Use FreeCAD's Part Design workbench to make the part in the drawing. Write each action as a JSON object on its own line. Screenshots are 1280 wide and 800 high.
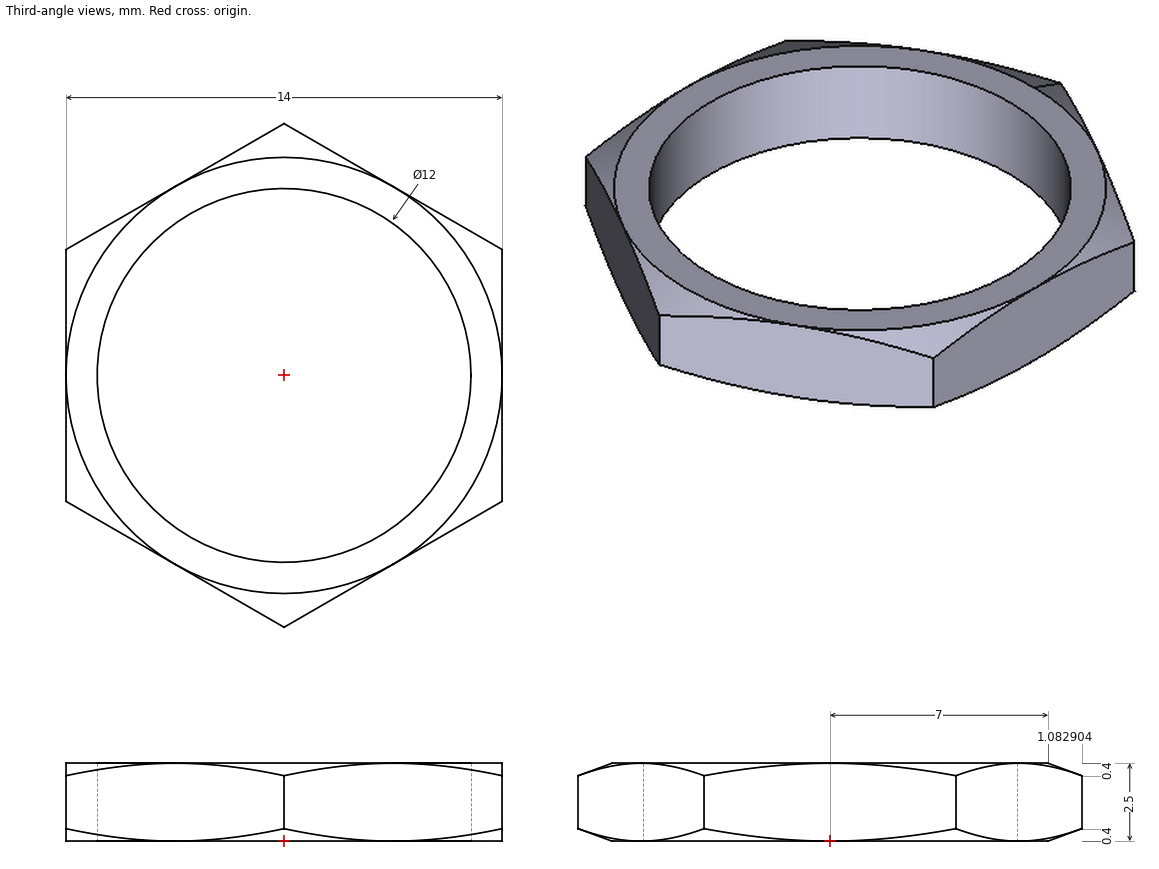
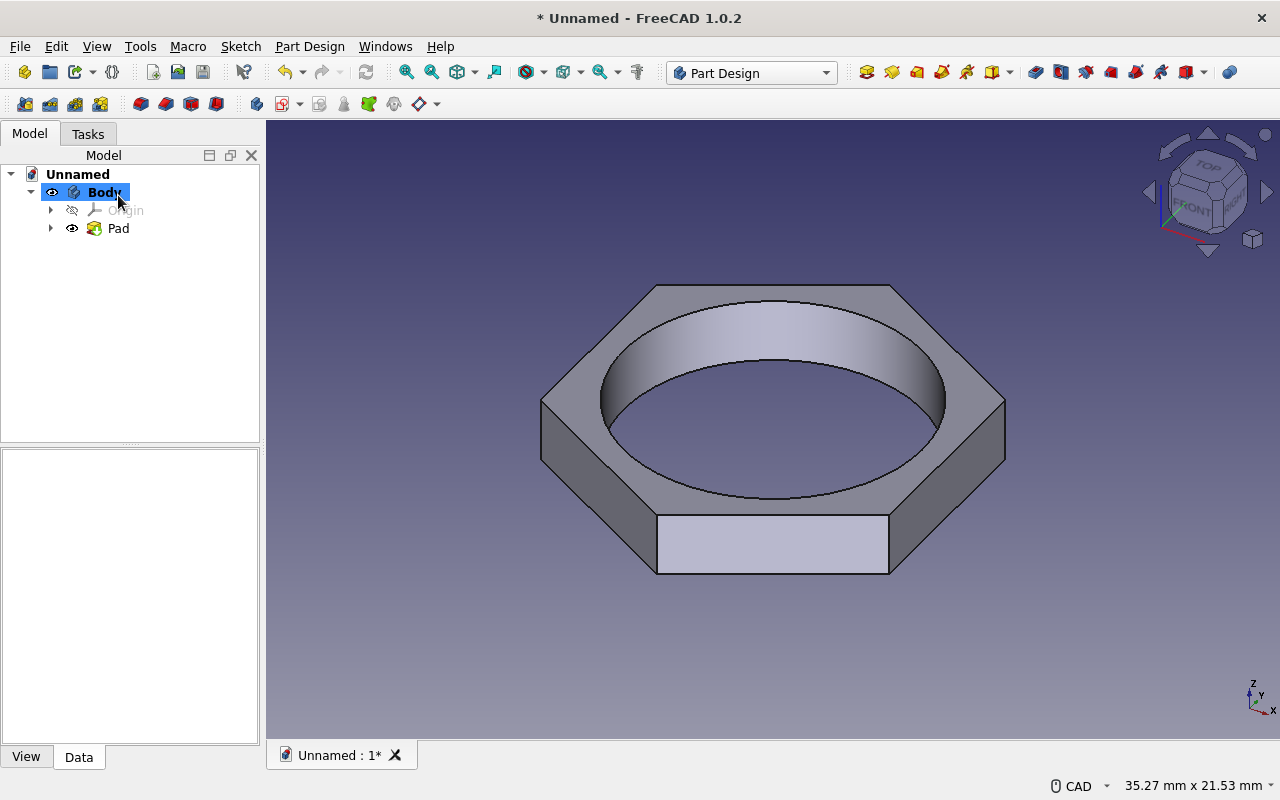
{"action": "left_click", "coordinate": [282, 104]}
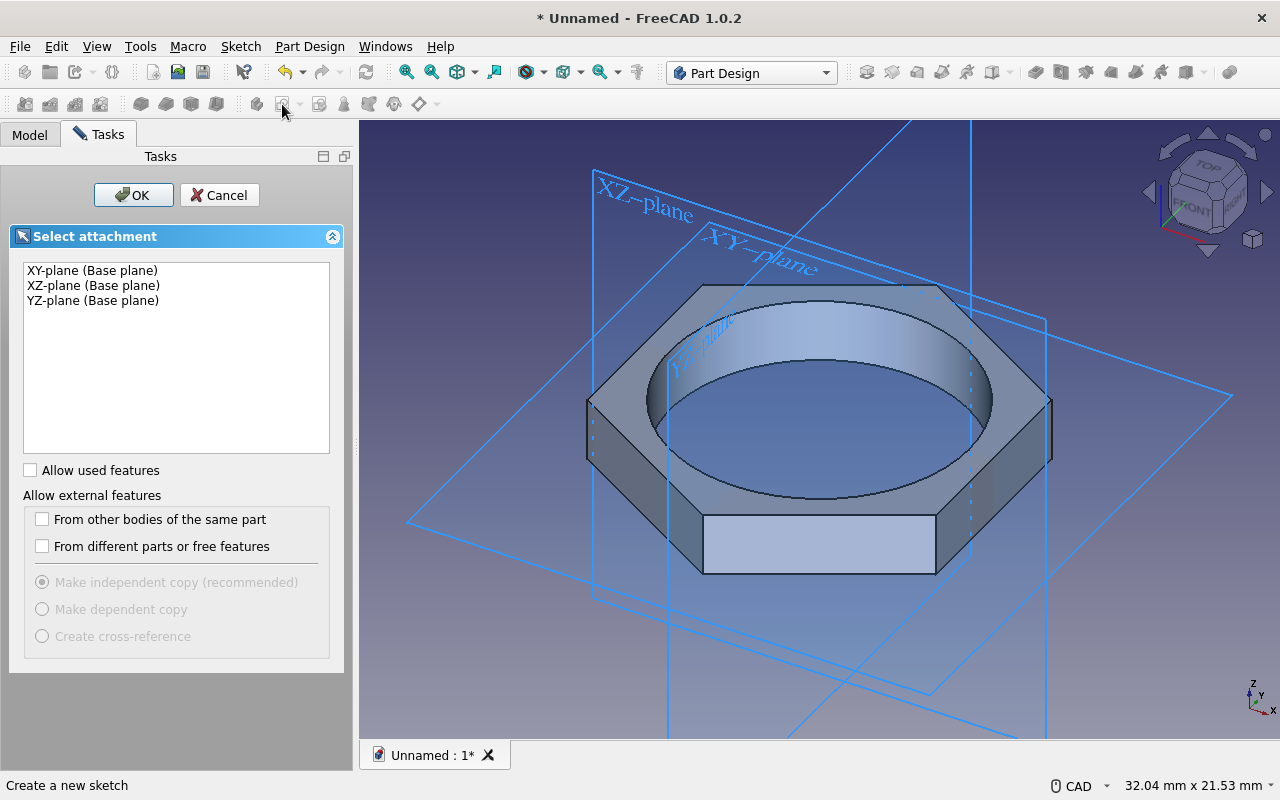
{"action": "left_click", "coordinate": [84, 300]}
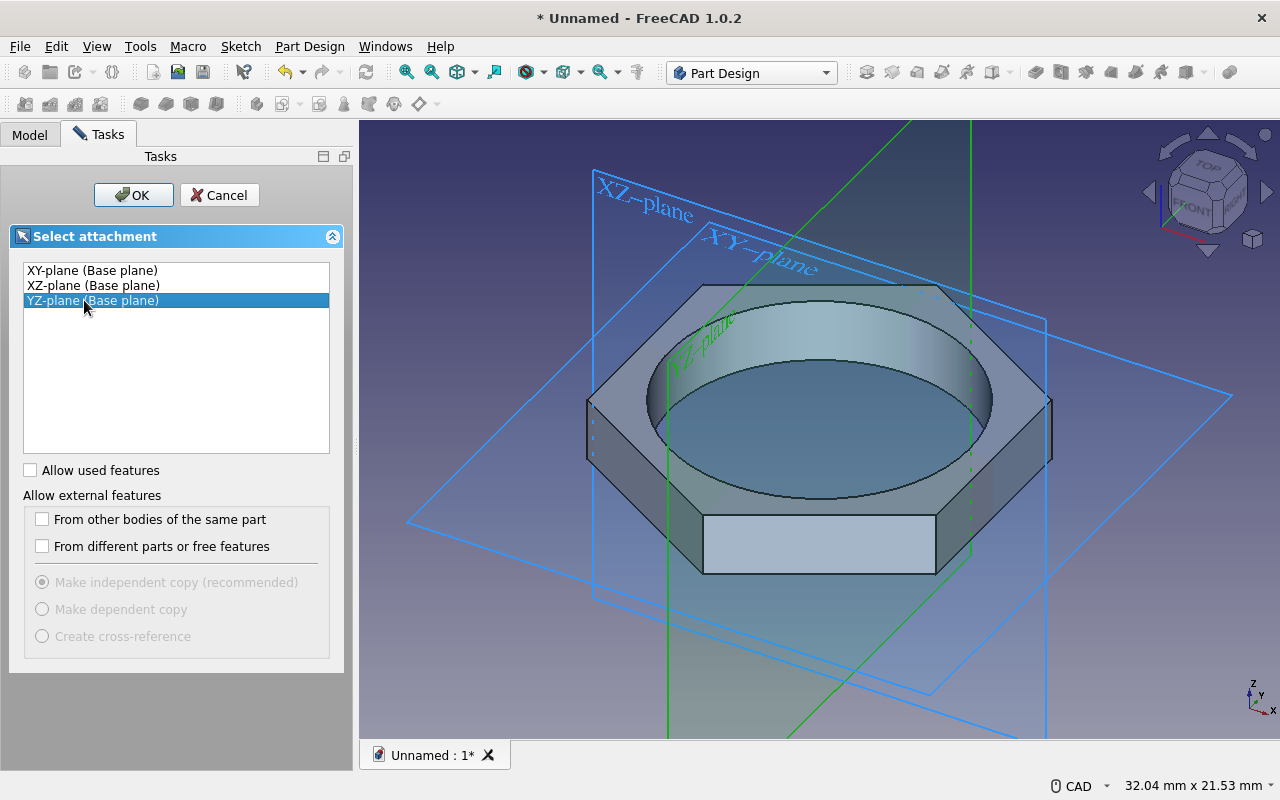
{"action": "left_click", "coordinate": [134, 195]}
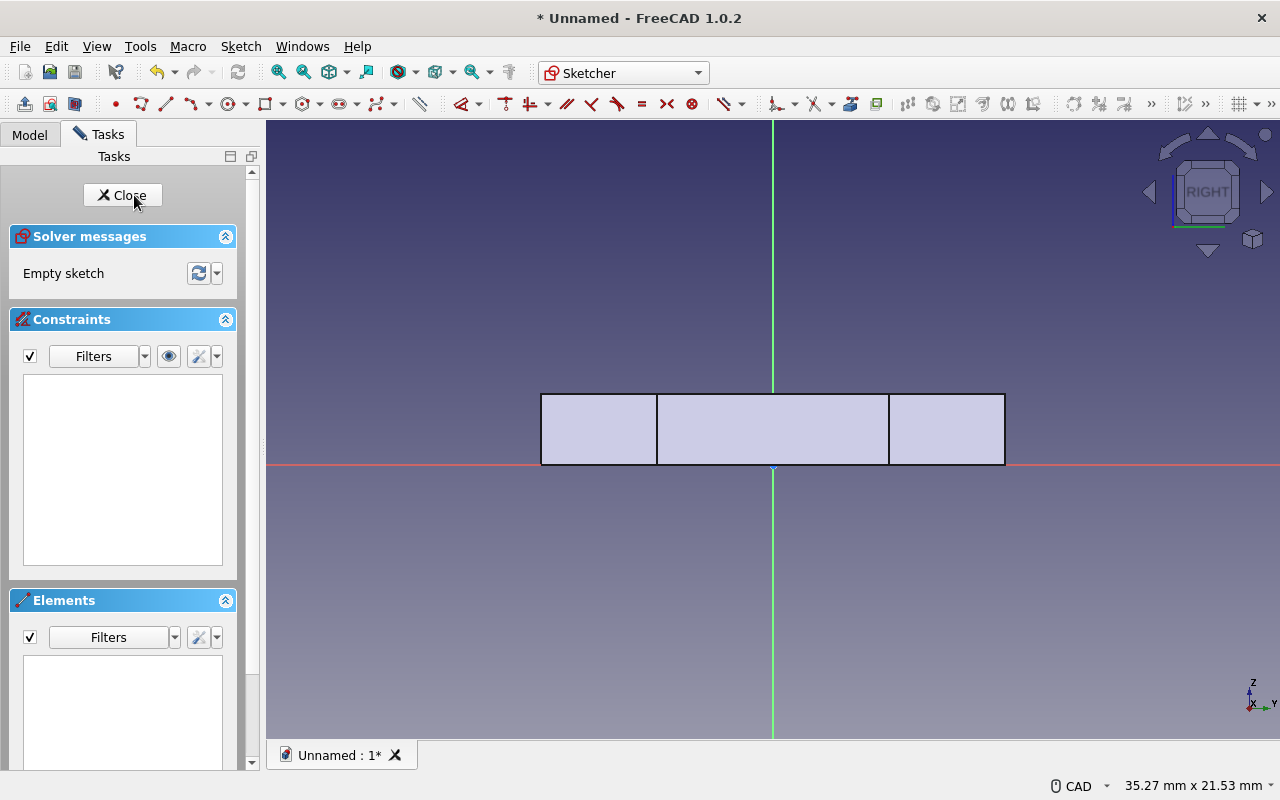
{"action": "key", "text": "q s"}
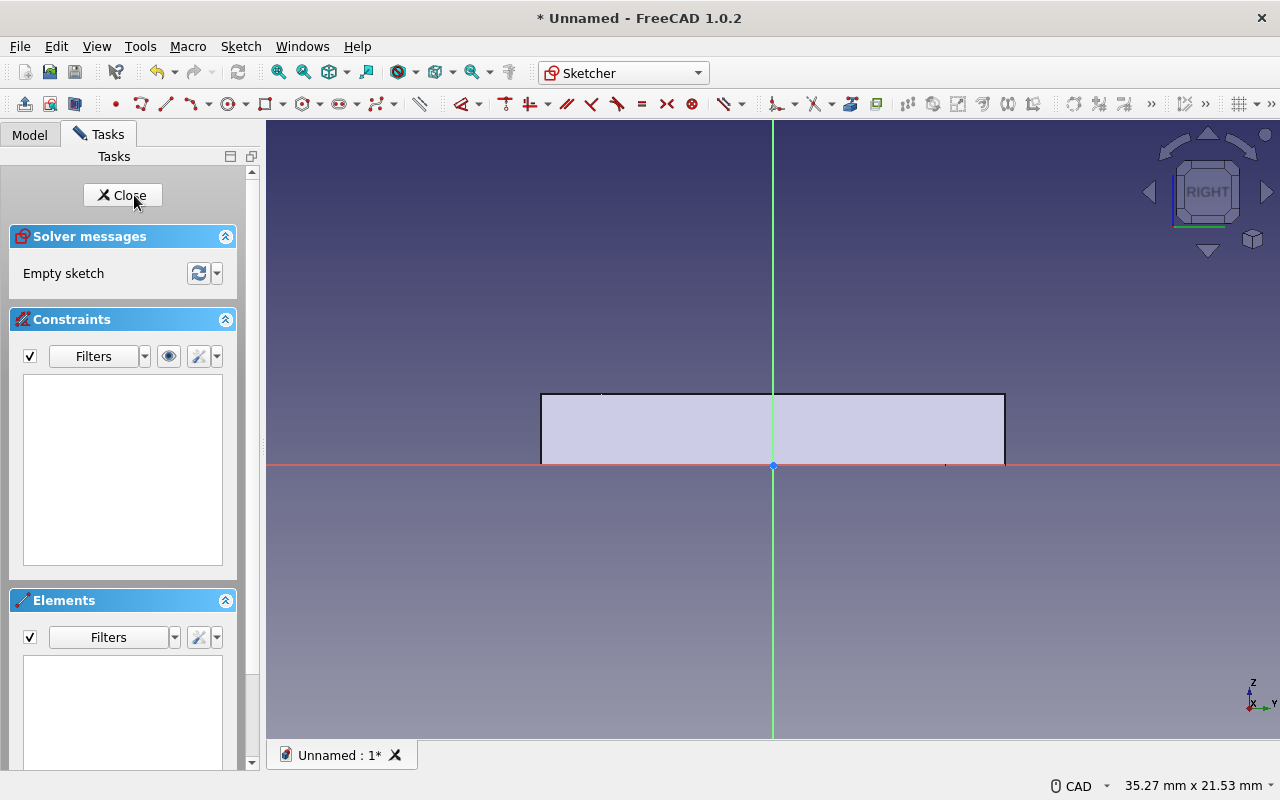
{"action": "scroll", "coordinate": [1046, 430], "scroll_direction": "up", "scroll_amount": 9}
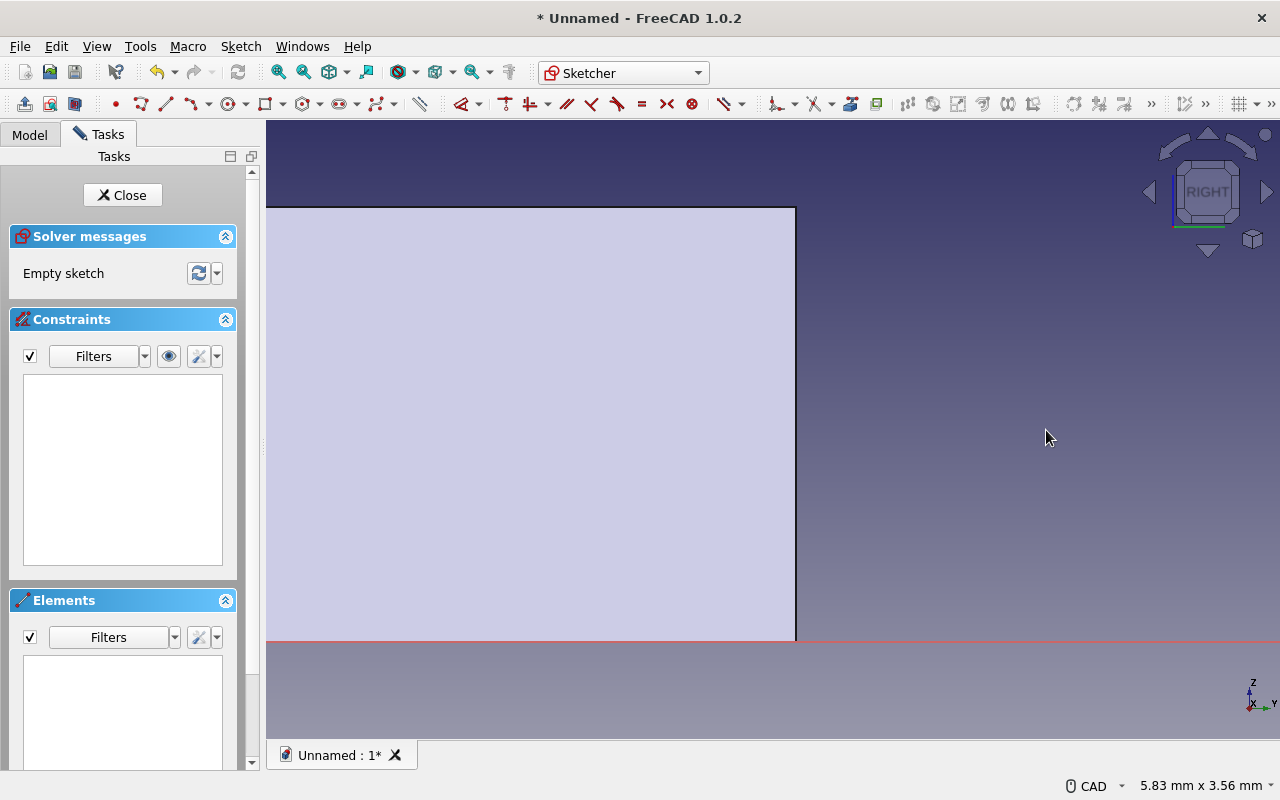
{"action": "key", "text": "g m"}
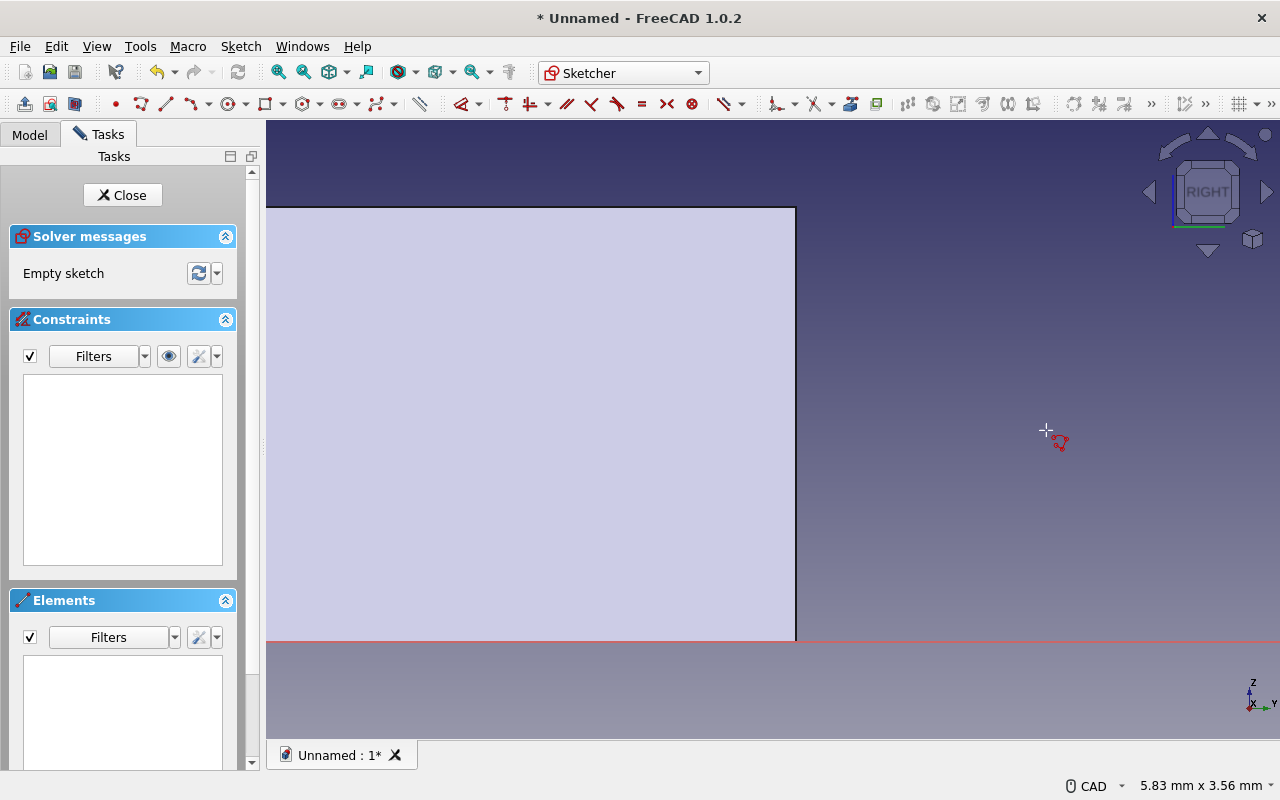
{"action": "left_click", "coordinate": [608, 207]}
{"action": "left_click", "coordinate": [796, 277]}
{"action": "left_click", "coordinate": [796, 207]}
{"action": "left_click", "coordinate": [608, 208]}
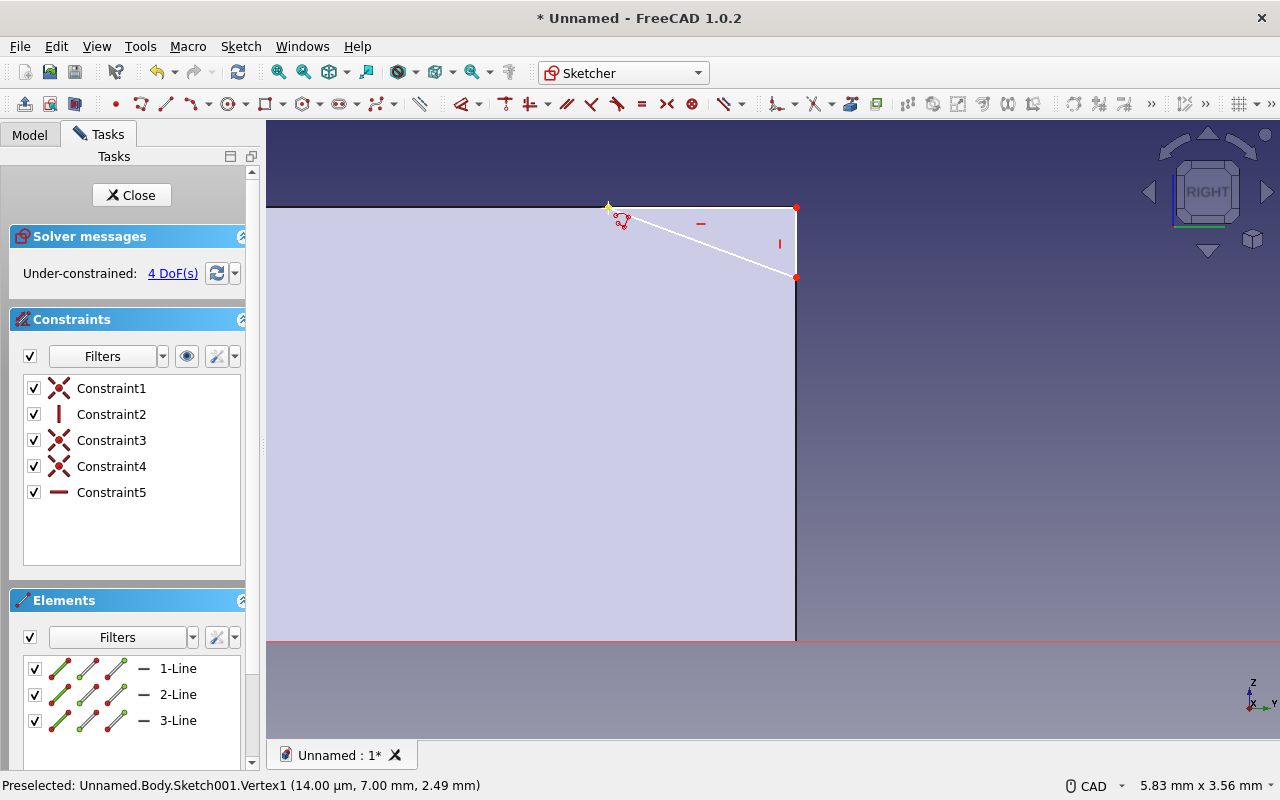
{"action": "left_click", "coordinate": [608, 642]}
{"action": "left_click", "coordinate": [796, 633]}
{"action": "left_click", "coordinate": [796, 572]}
{"action": "left_click", "coordinate": [608, 642]}
{"action": "key", "text": "Escape"}
{"action": "key", "text": "Escape"}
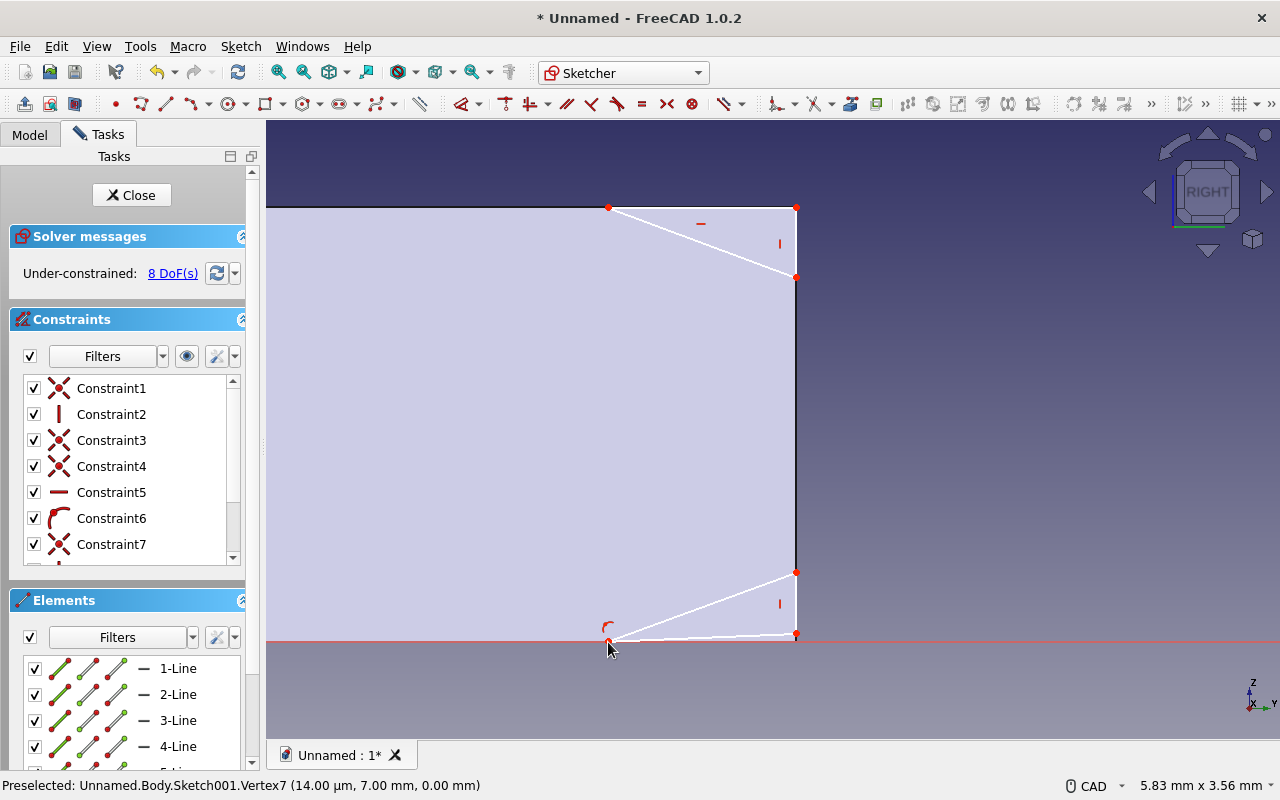
{"action": "left_click", "coordinate": [664, 639]}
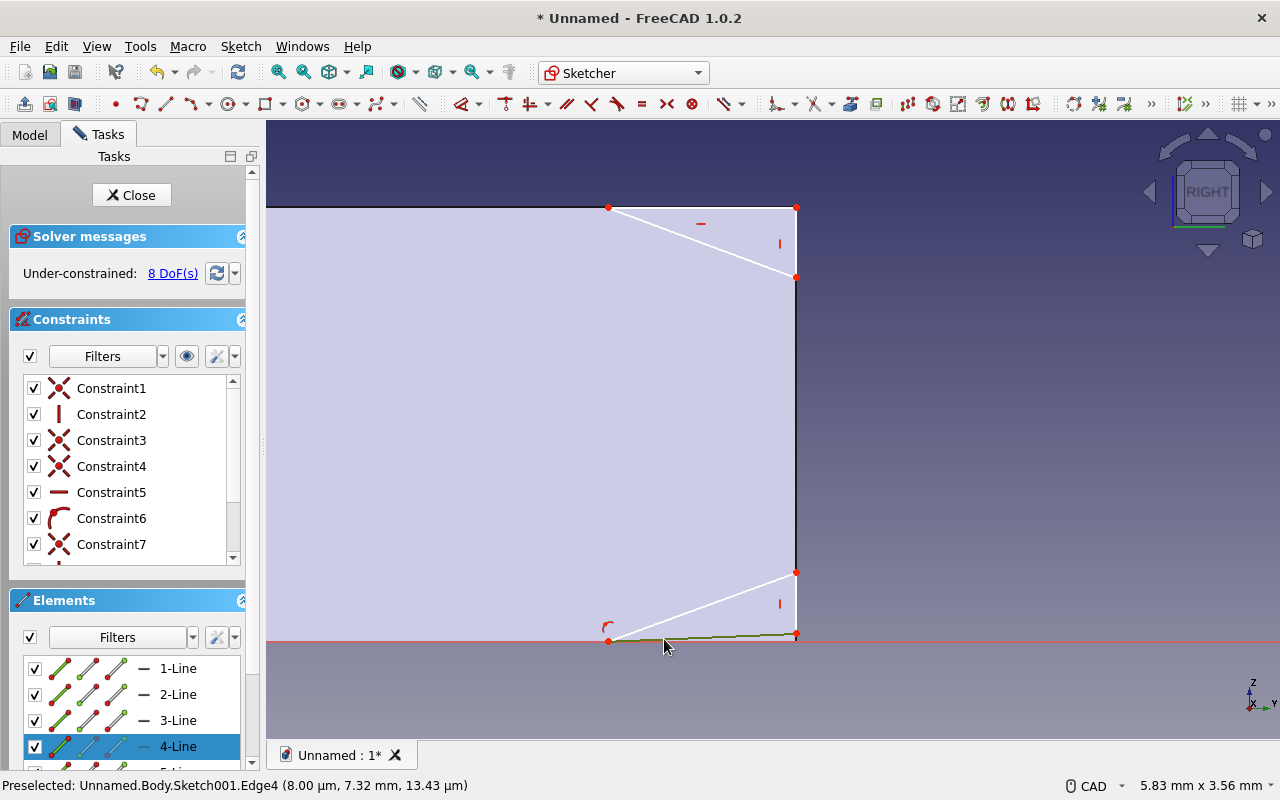
{"action": "key", "text": "h"}